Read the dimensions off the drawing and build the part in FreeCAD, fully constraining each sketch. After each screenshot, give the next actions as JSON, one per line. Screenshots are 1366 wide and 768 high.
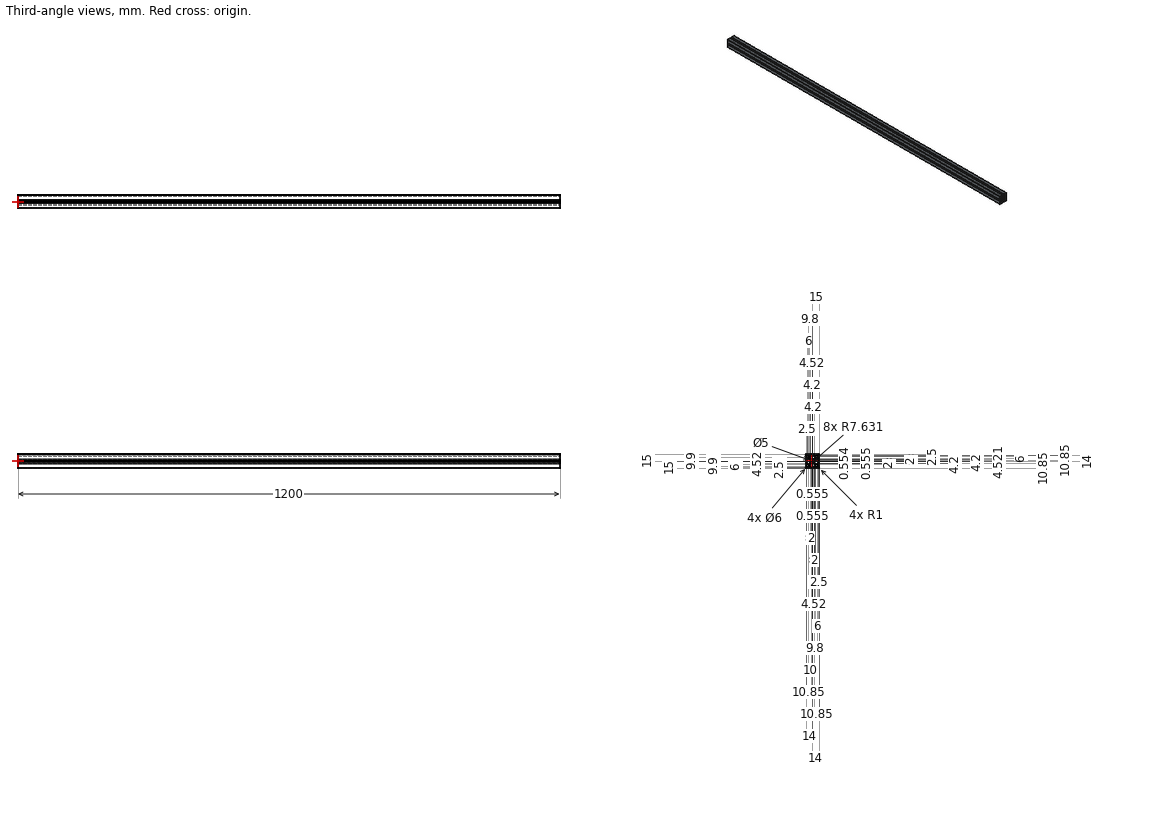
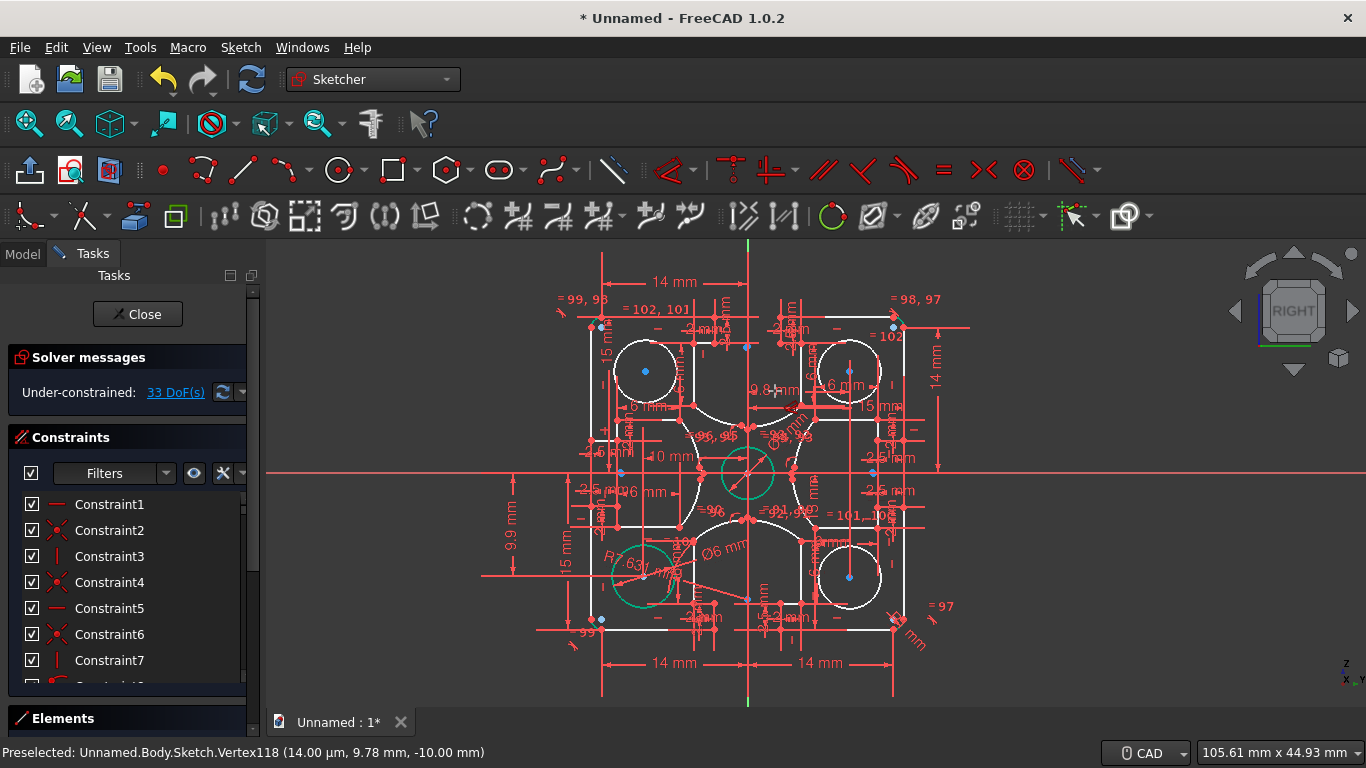
{"action": "left_click", "coordinate": [850, 578]}
{"action": "left_click", "coordinate": [932, 549]}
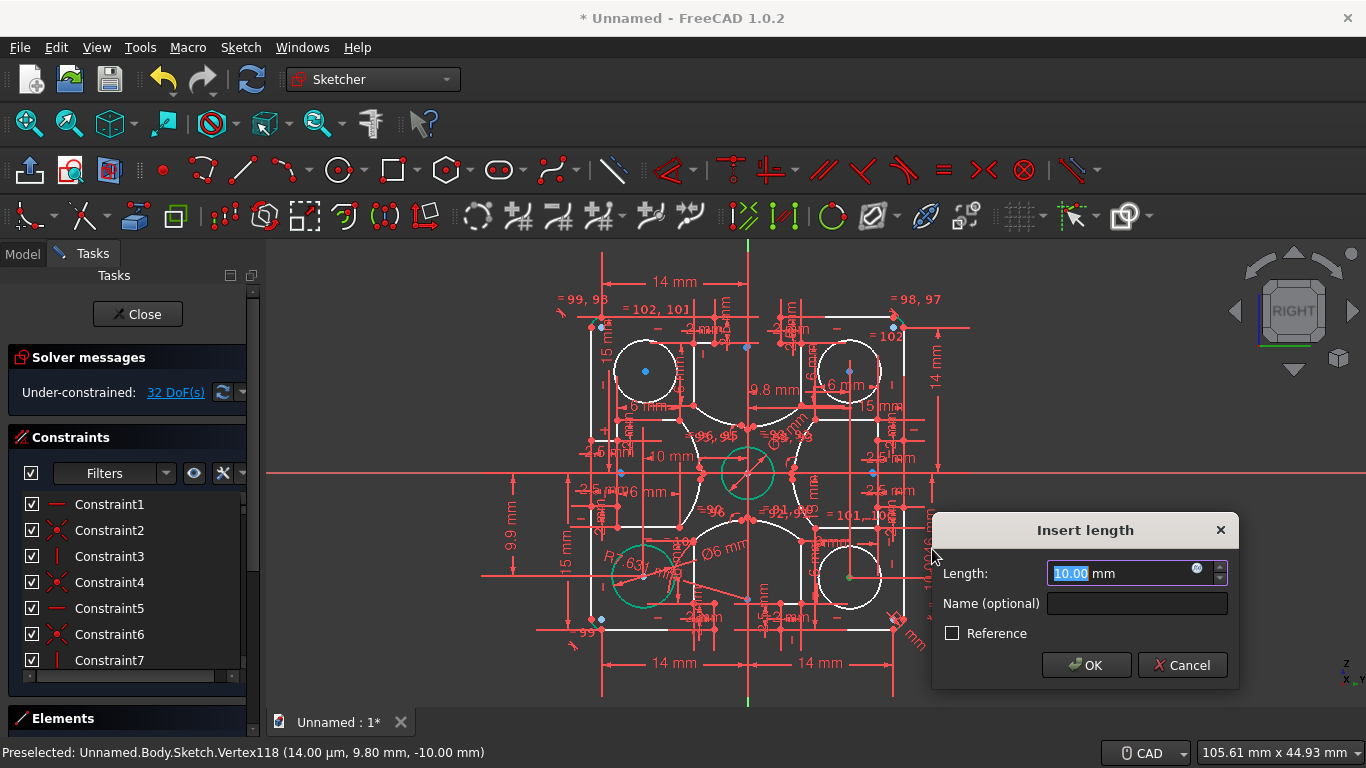
{"action": "type", "text": "9.9"}
{"action": "key", "text": "Return"}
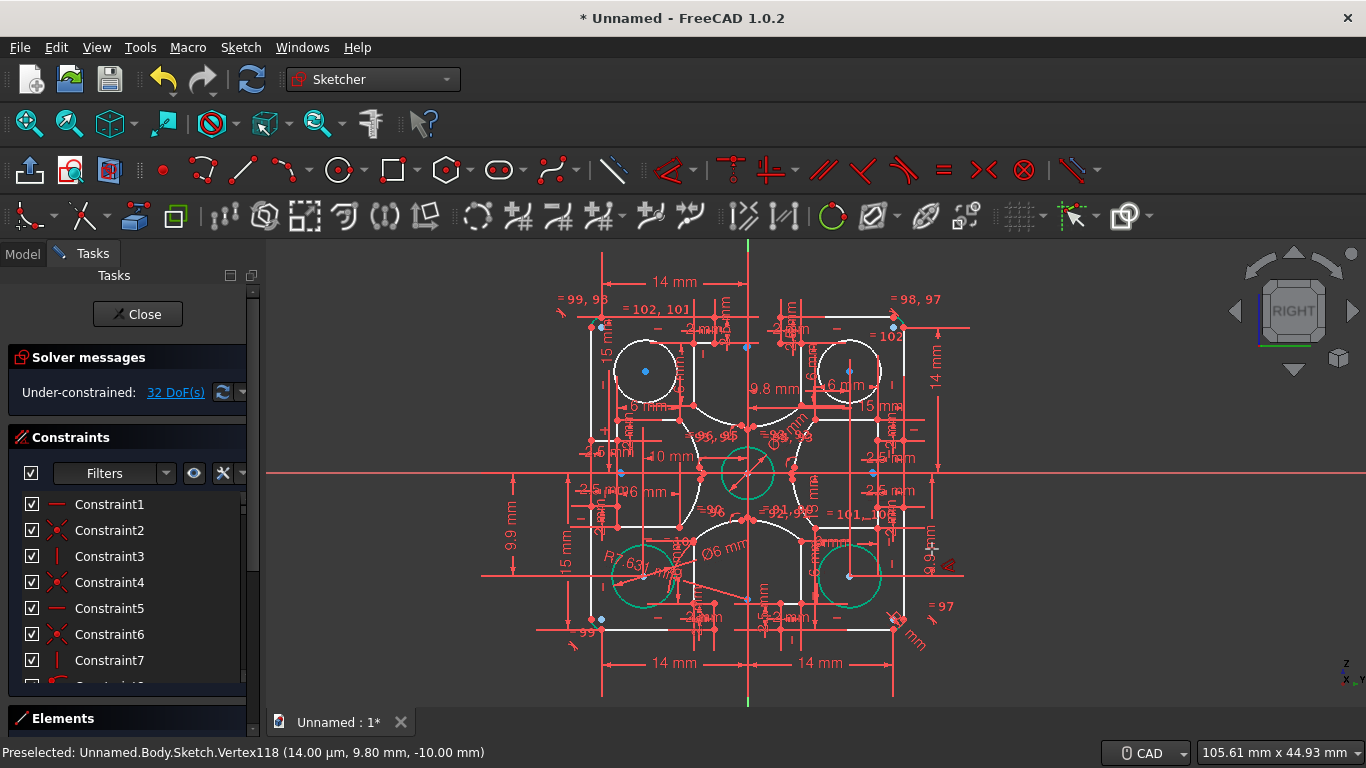
{"action": "left_click", "coordinate": [646, 372]}
{"action": "left_click", "coordinate": [720, 507]}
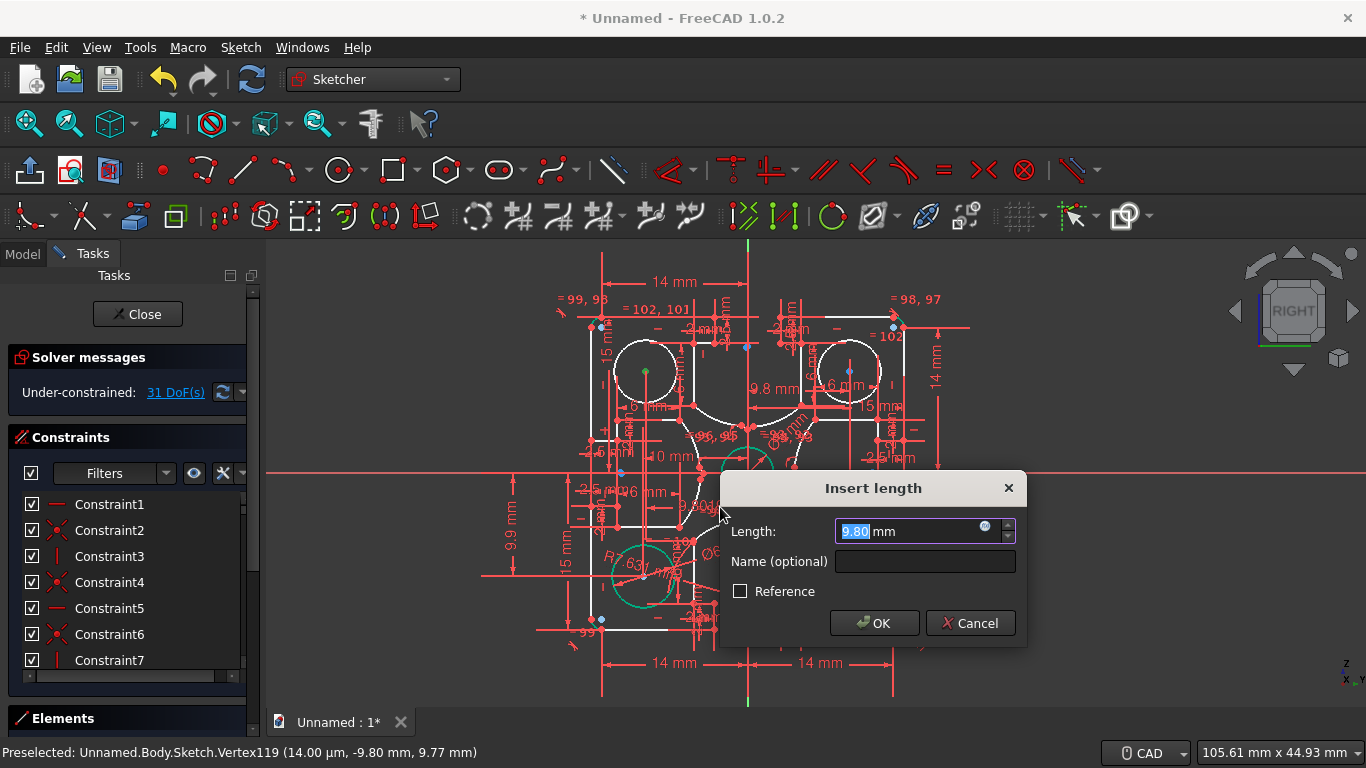
{"action": "type", "text": "9.8"}
{"action": "key", "text": "Return"}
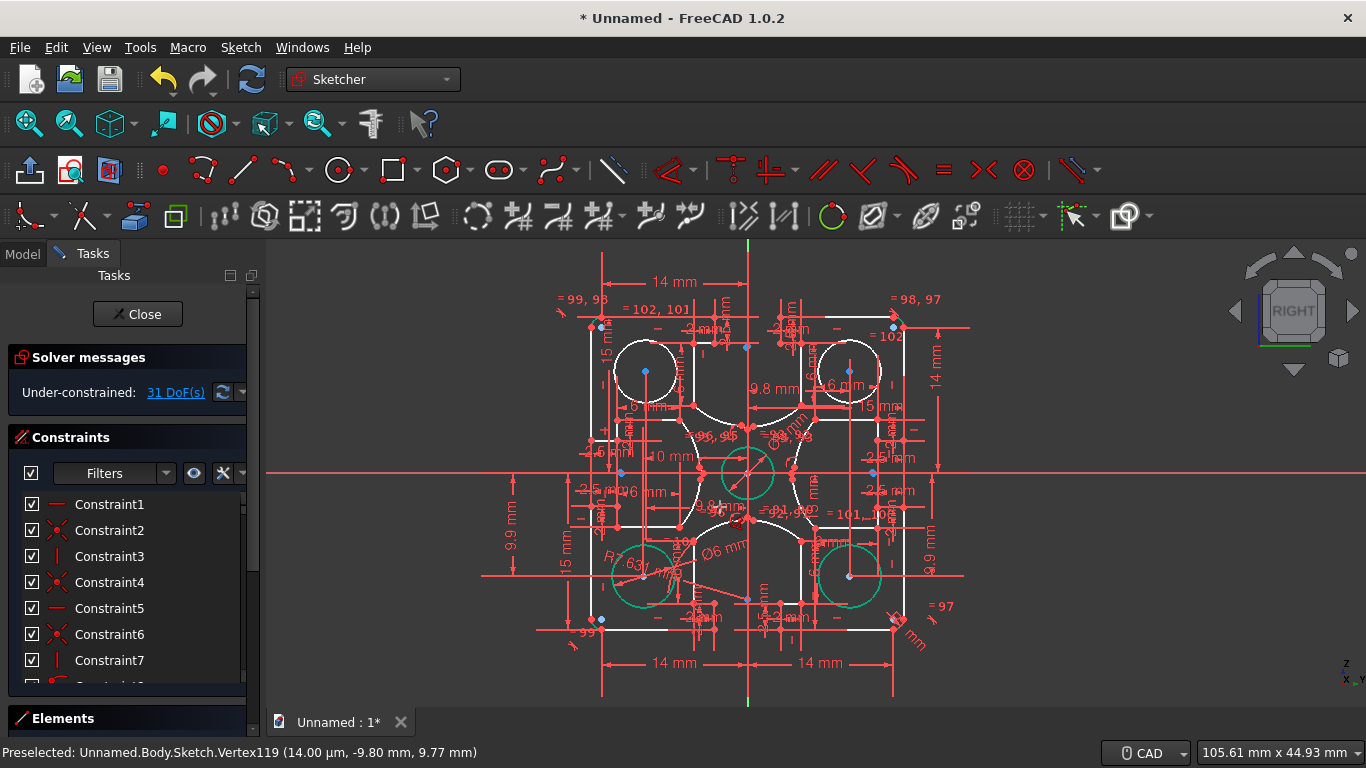
{"action": "left_click", "coordinate": [646, 372]}
{"action": "left_click", "coordinate": [564, 399]}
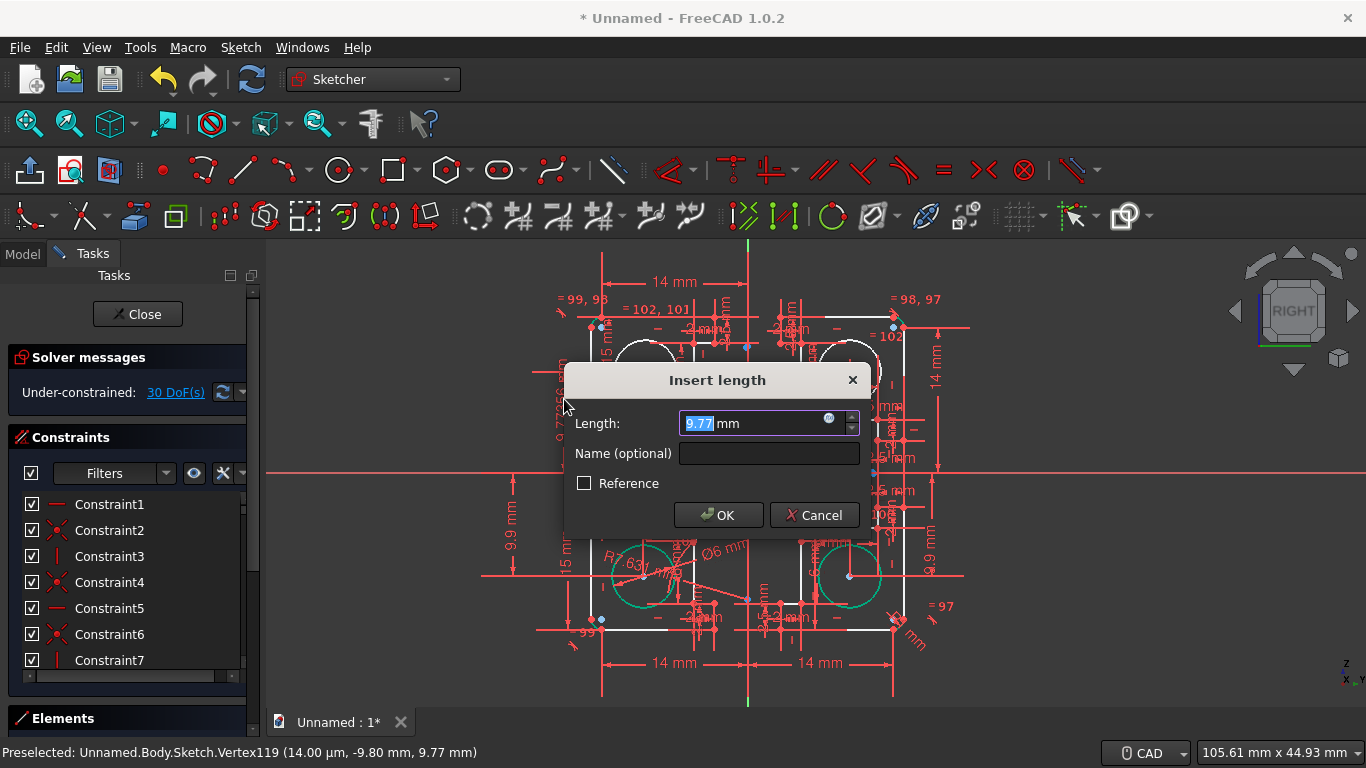
{"action": "type", "text": "9.9"}
{"action": "key", "text": "Return"}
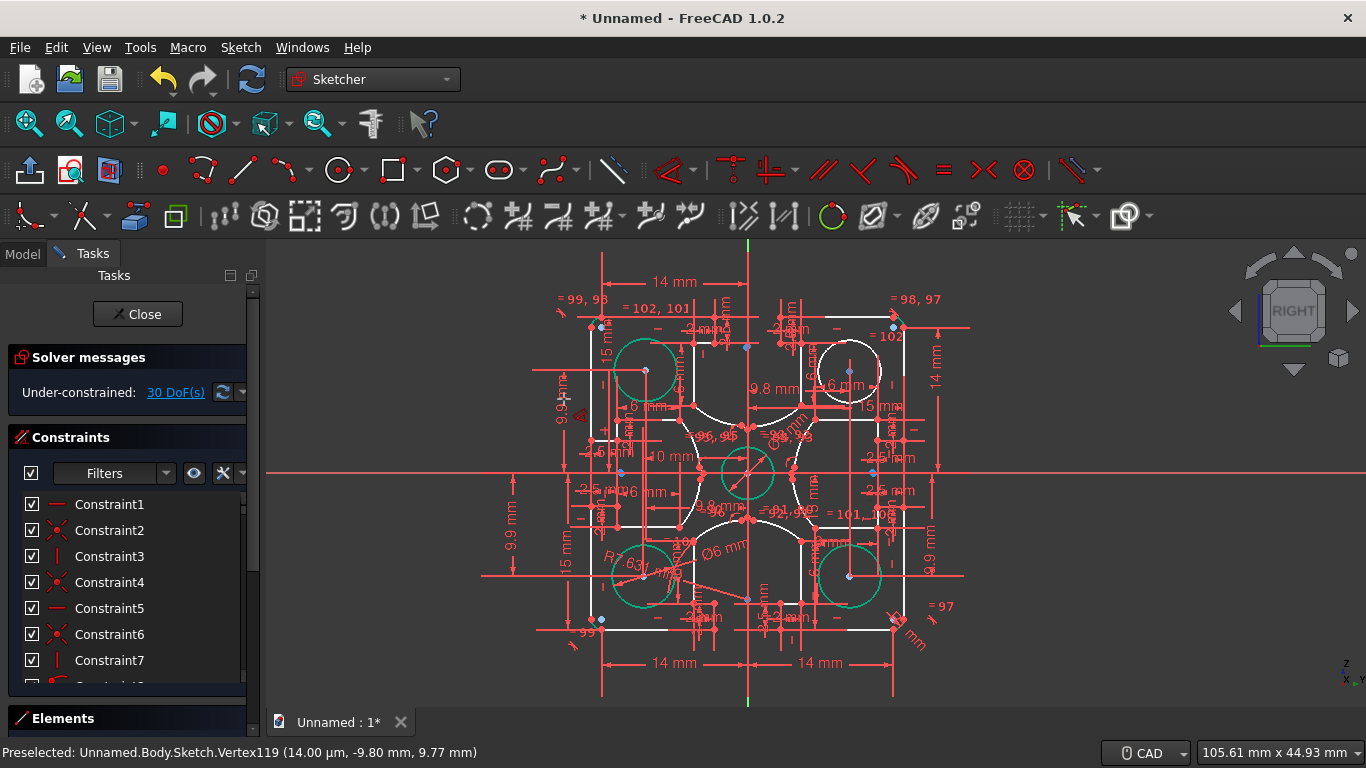
{"action": "left_click", "coordinate": [850, 372]}
{"action": "left_click", "coordinate": [799, 290]}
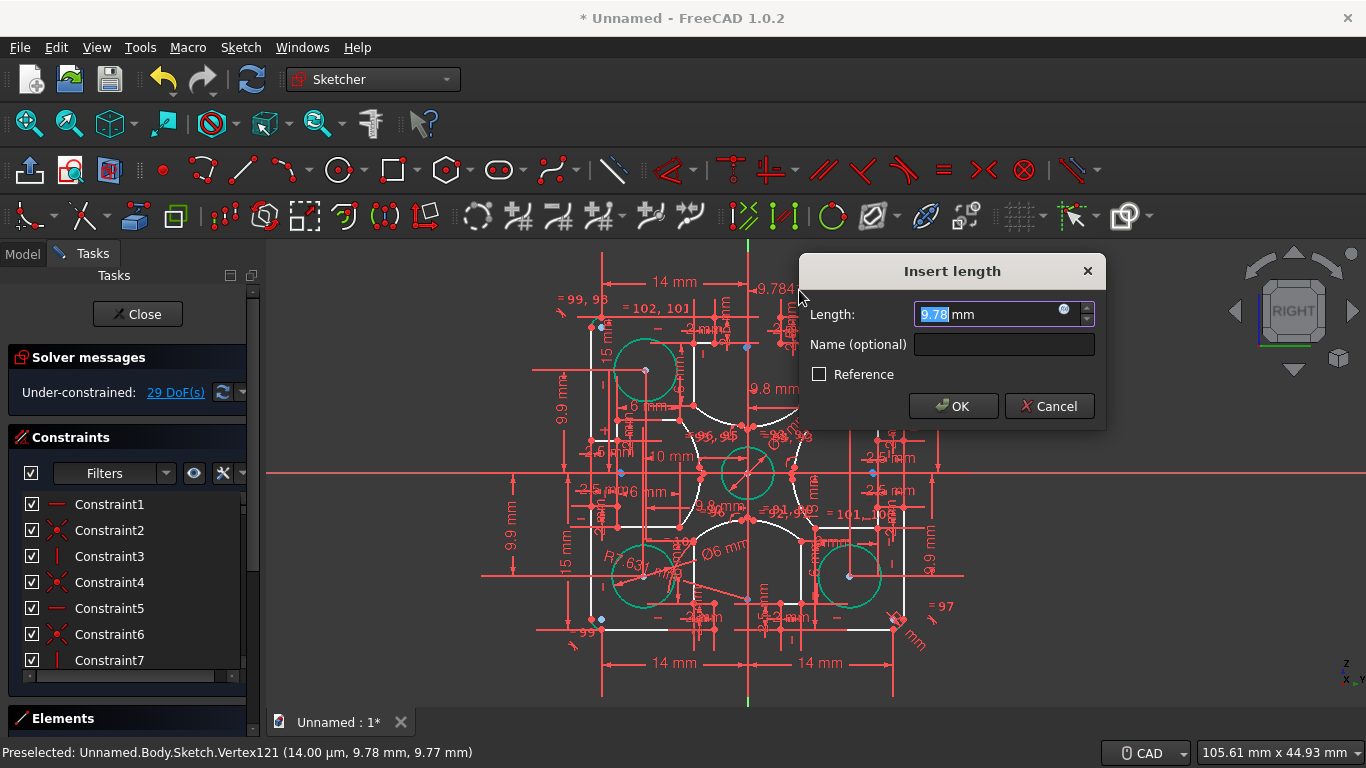
{"action": "type", "text": "9.8"}
{"action": "key", "text": "Return"}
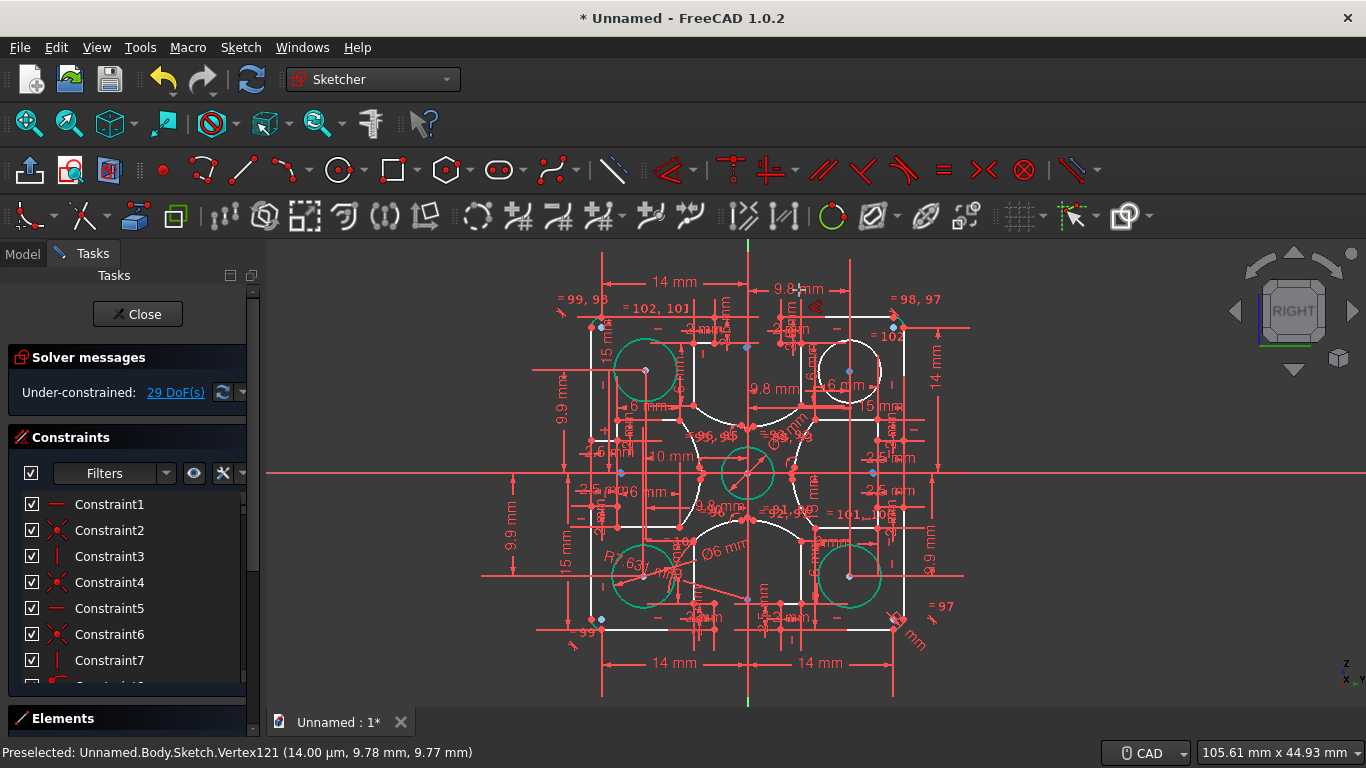
{"action": "left_click", "coordinate": [850, 372]}
{"action": "left_click", "coordinate": [956, 399]}